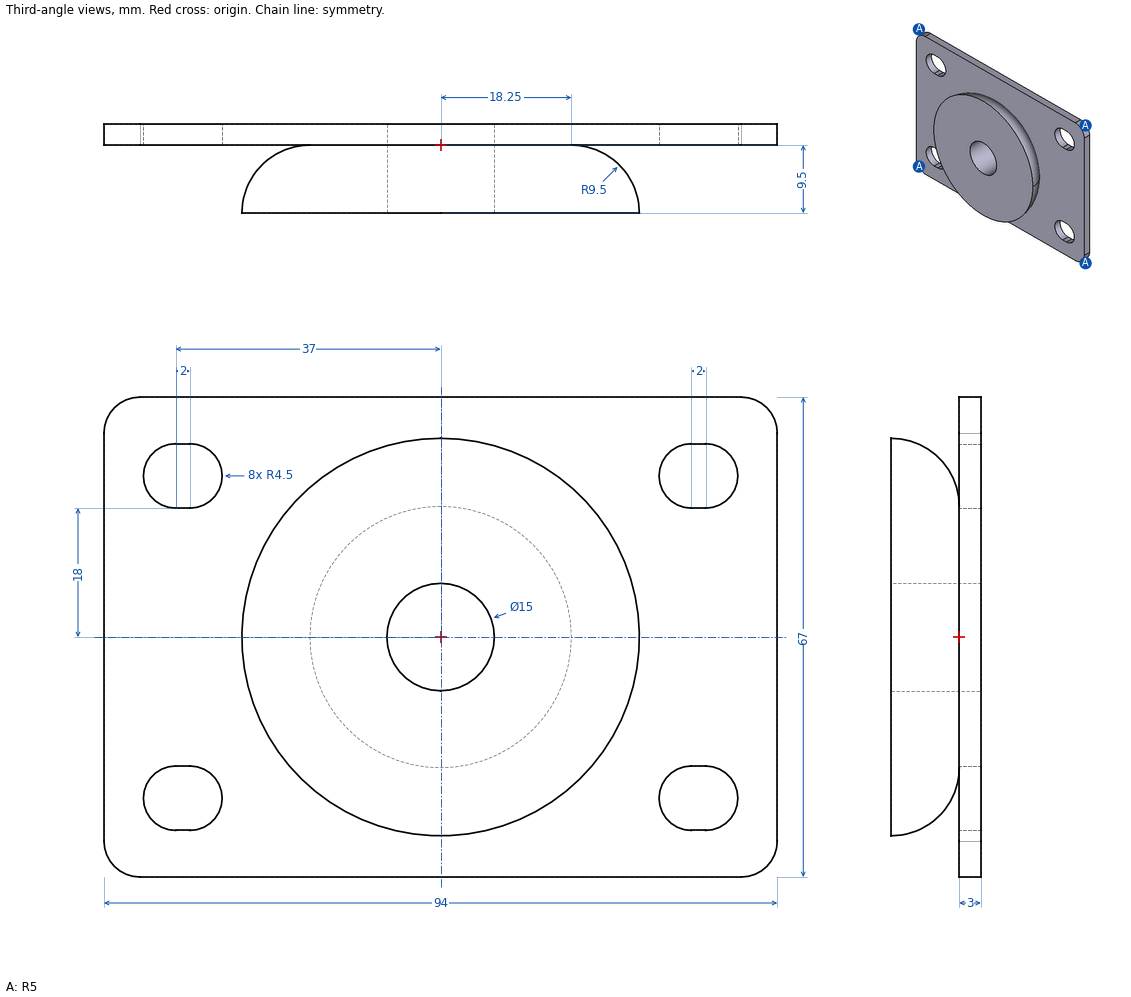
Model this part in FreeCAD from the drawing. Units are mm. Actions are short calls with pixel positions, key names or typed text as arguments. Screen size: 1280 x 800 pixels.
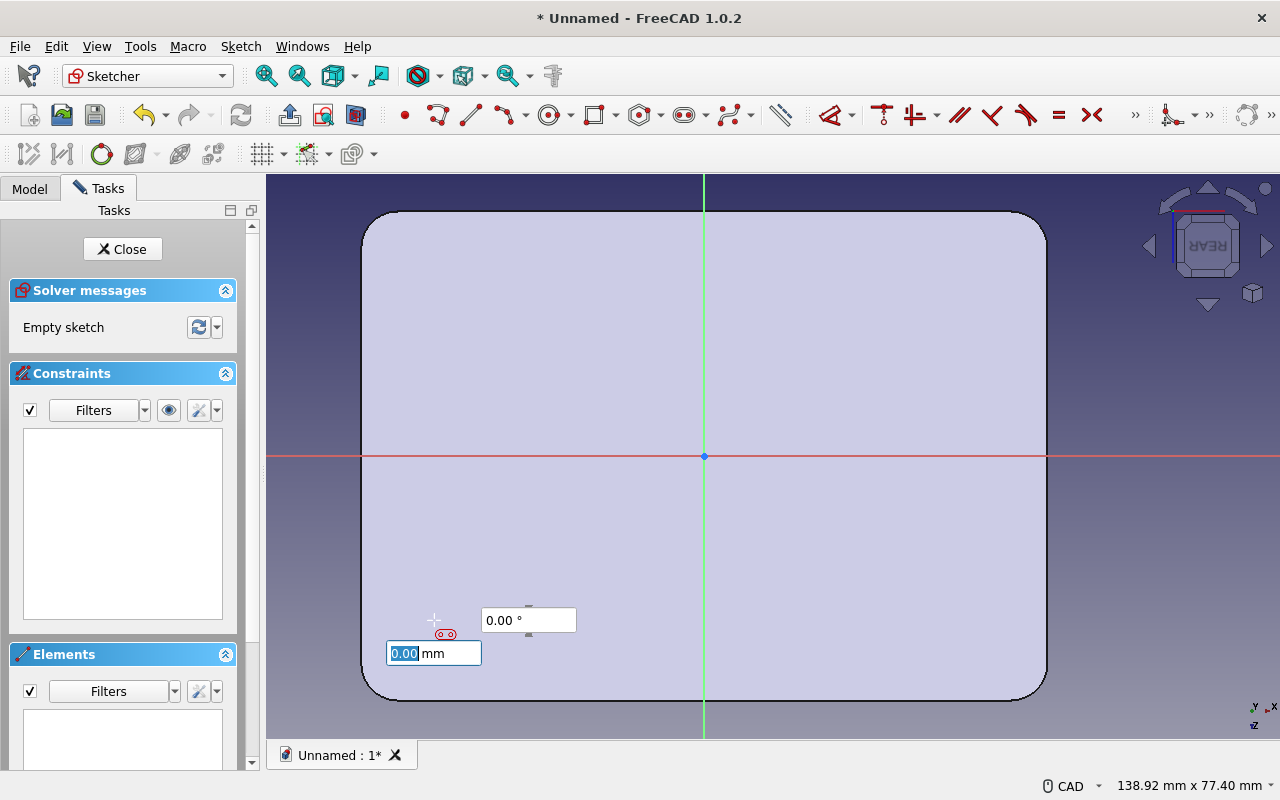
click(449, 620)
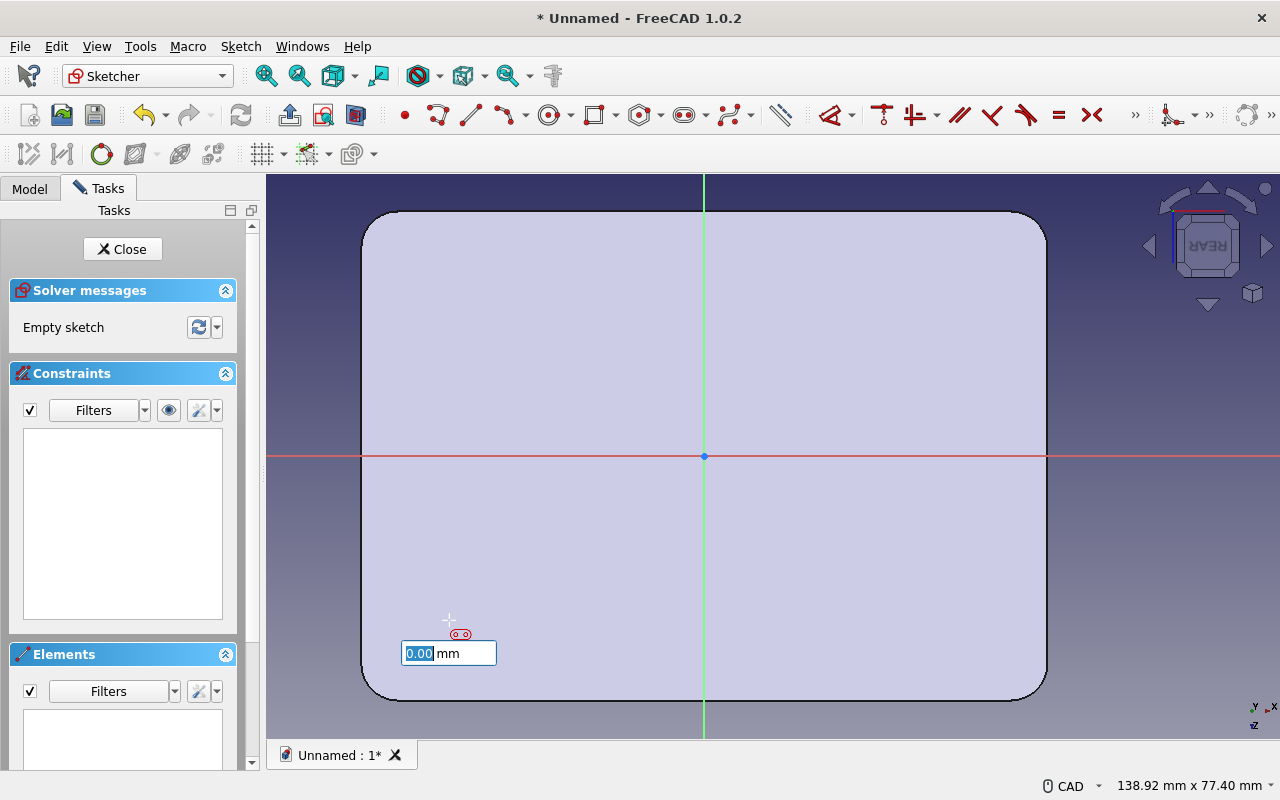
click(442, 653)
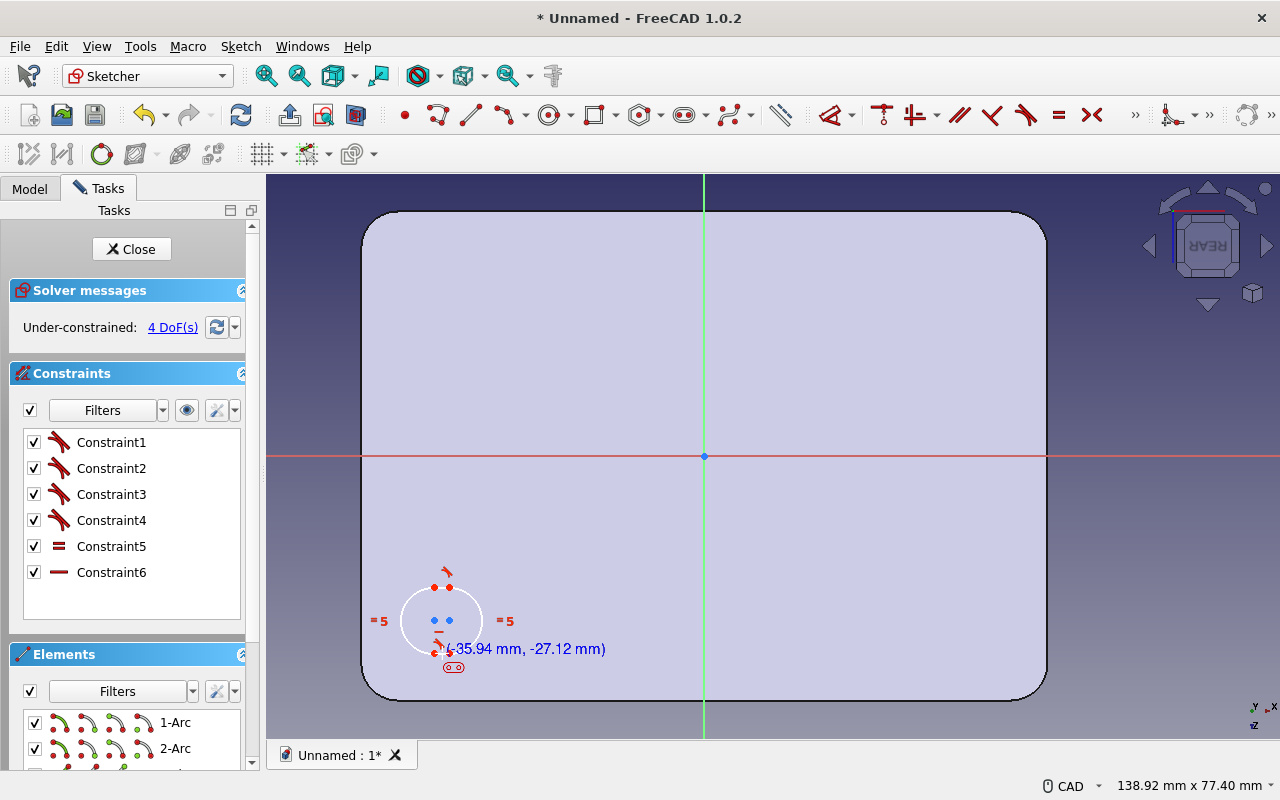
click(960, 620)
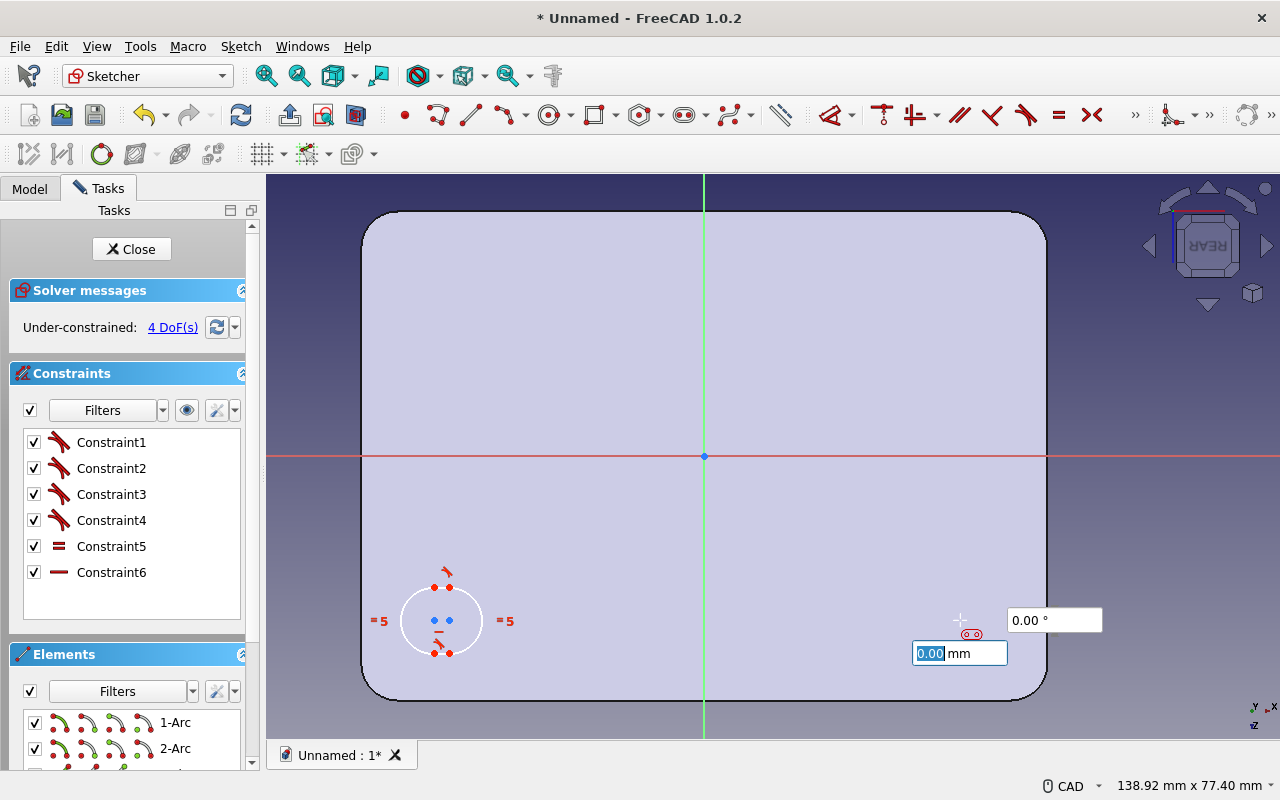
click(974, 620)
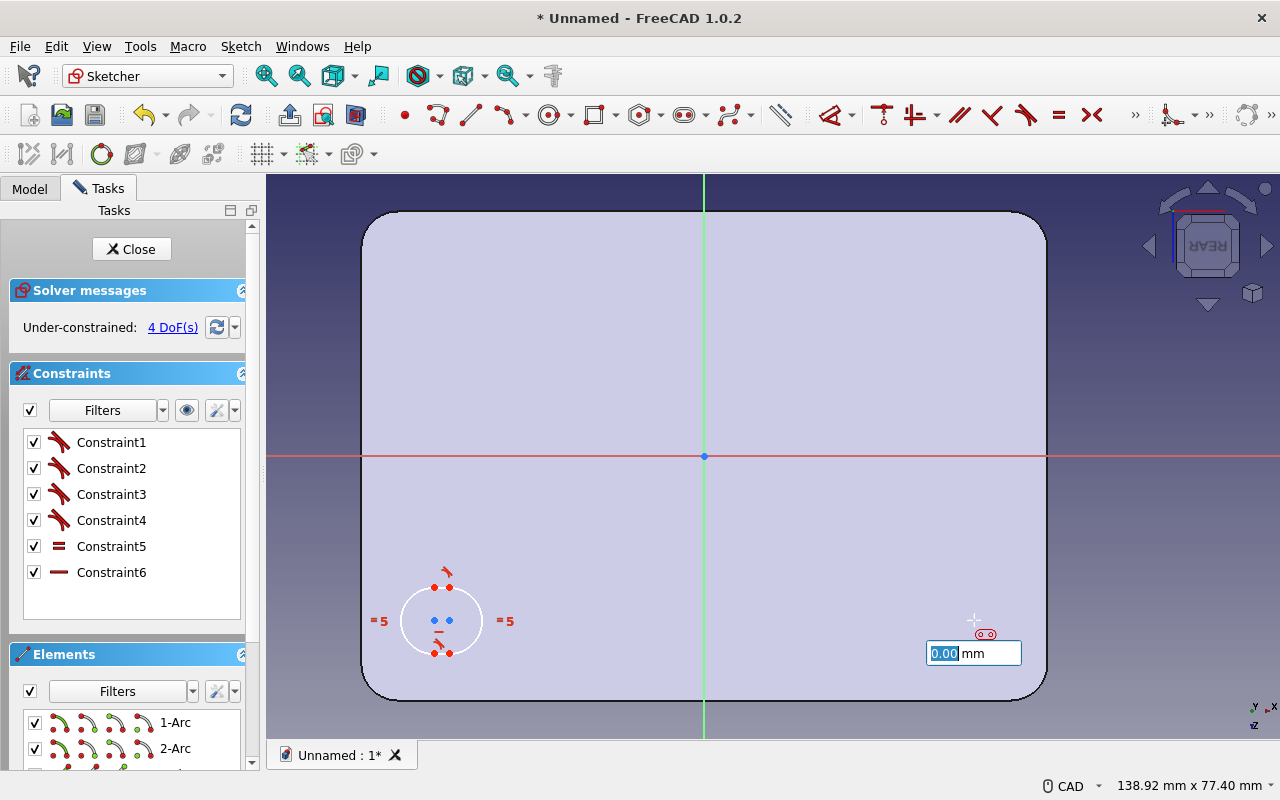
click(967, 587)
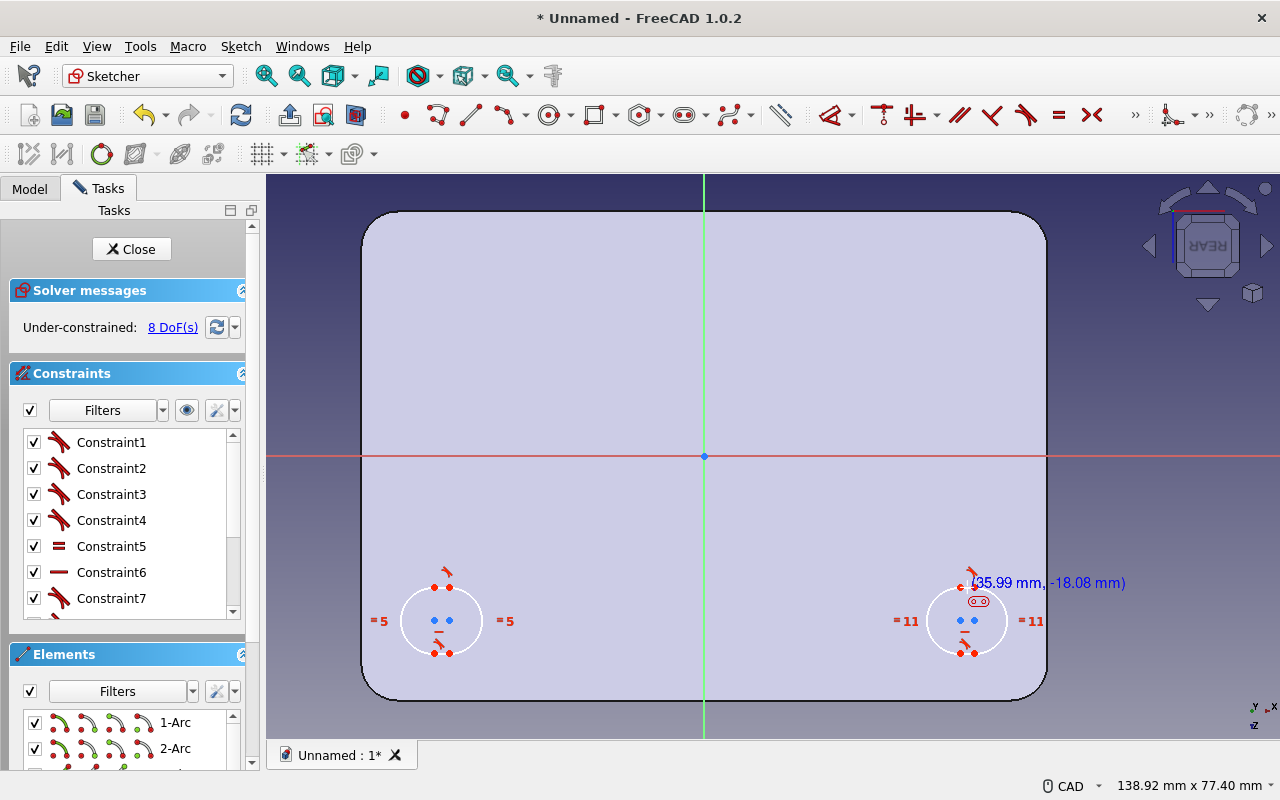
click(960, 292)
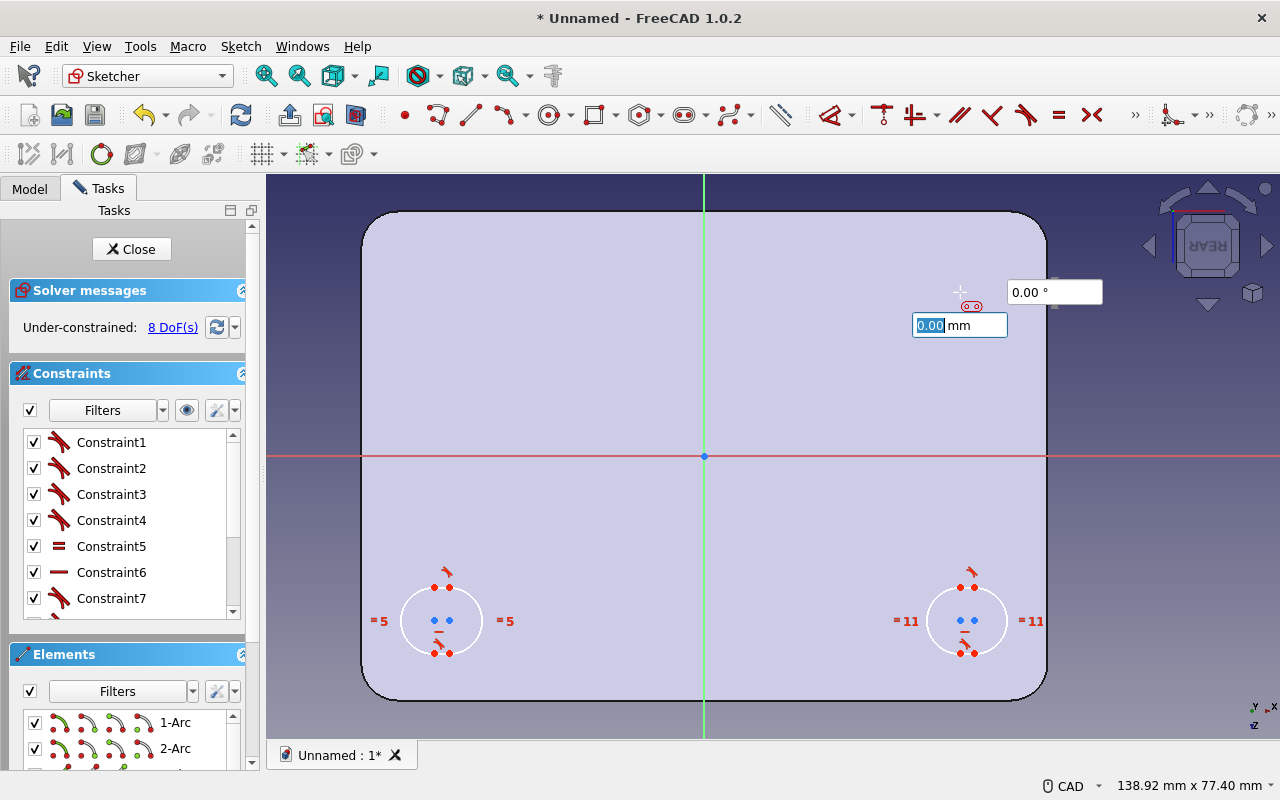
click(974, 292)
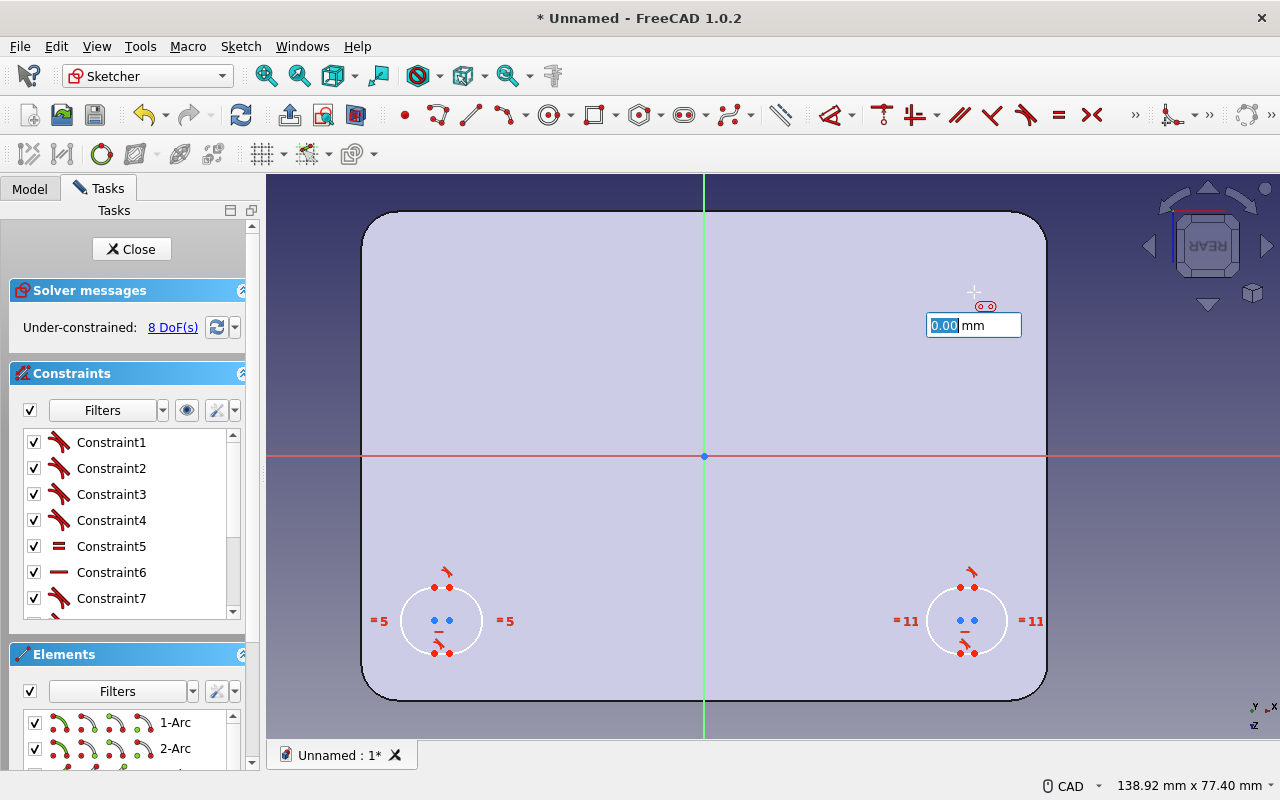
click(967, 259)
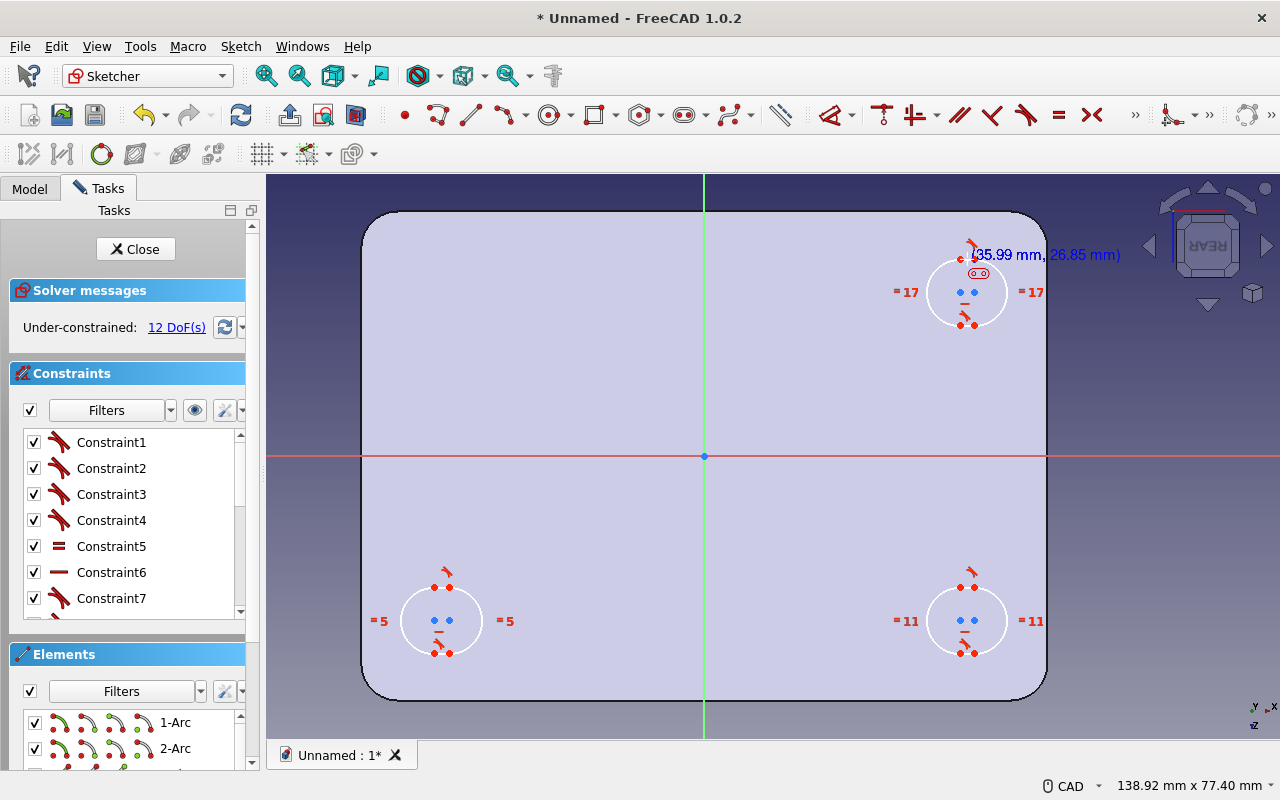
click(434, 292)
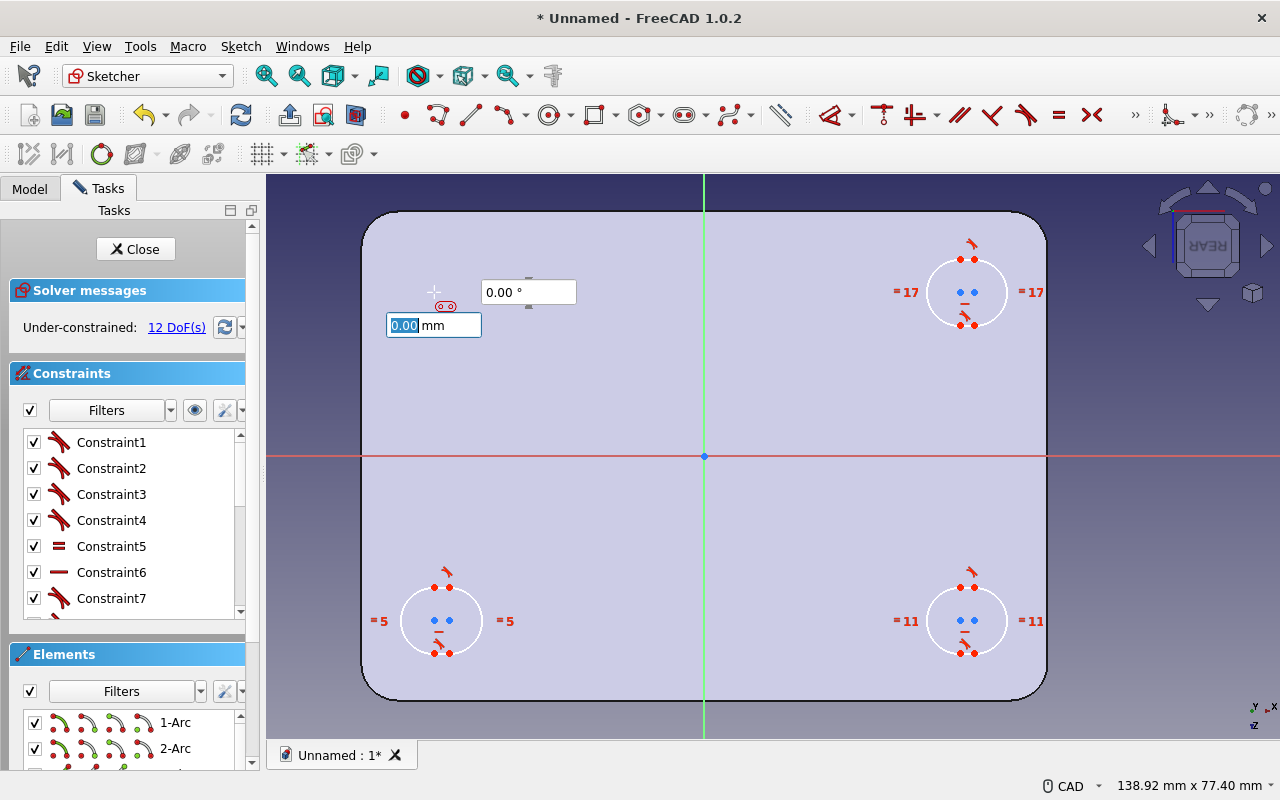
click(449, 292)